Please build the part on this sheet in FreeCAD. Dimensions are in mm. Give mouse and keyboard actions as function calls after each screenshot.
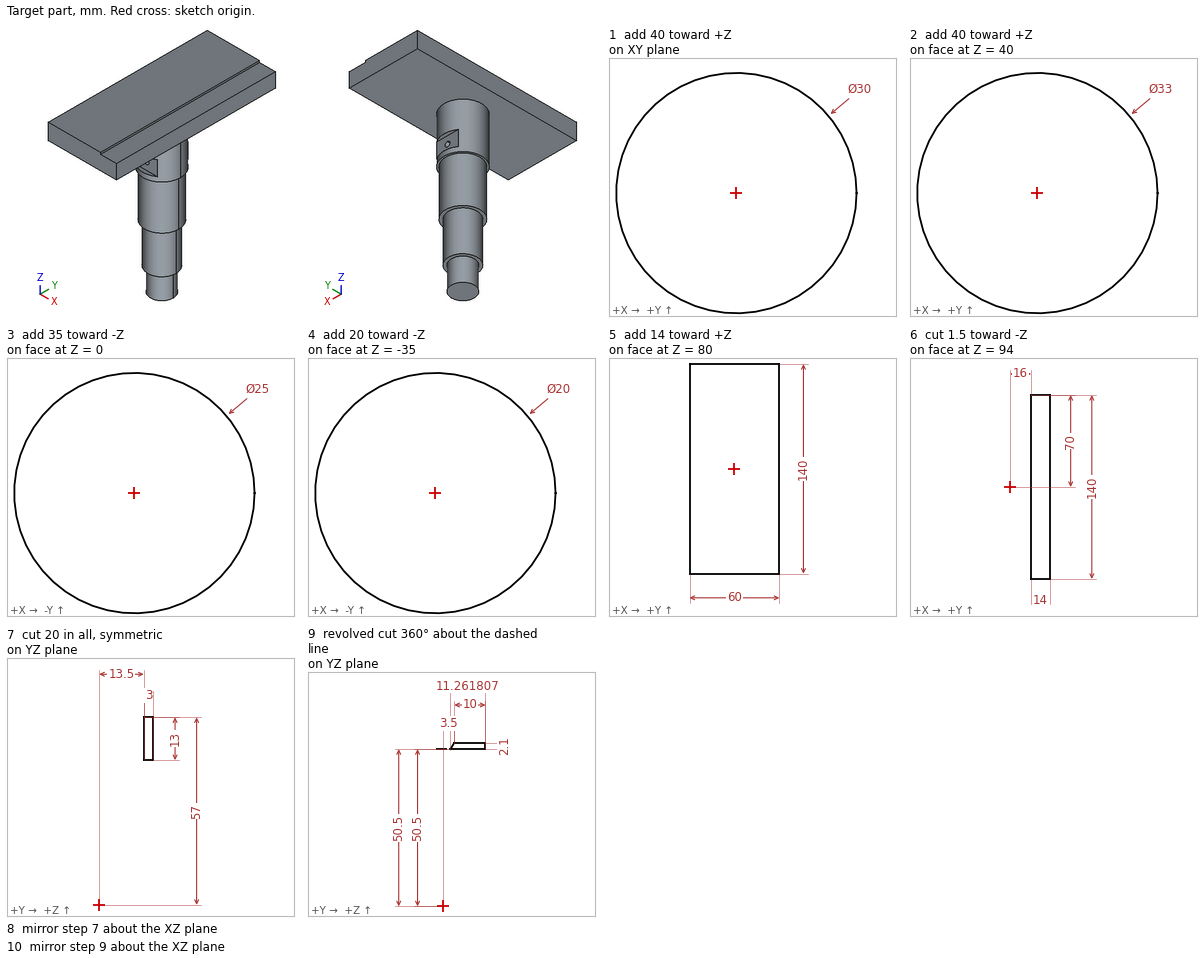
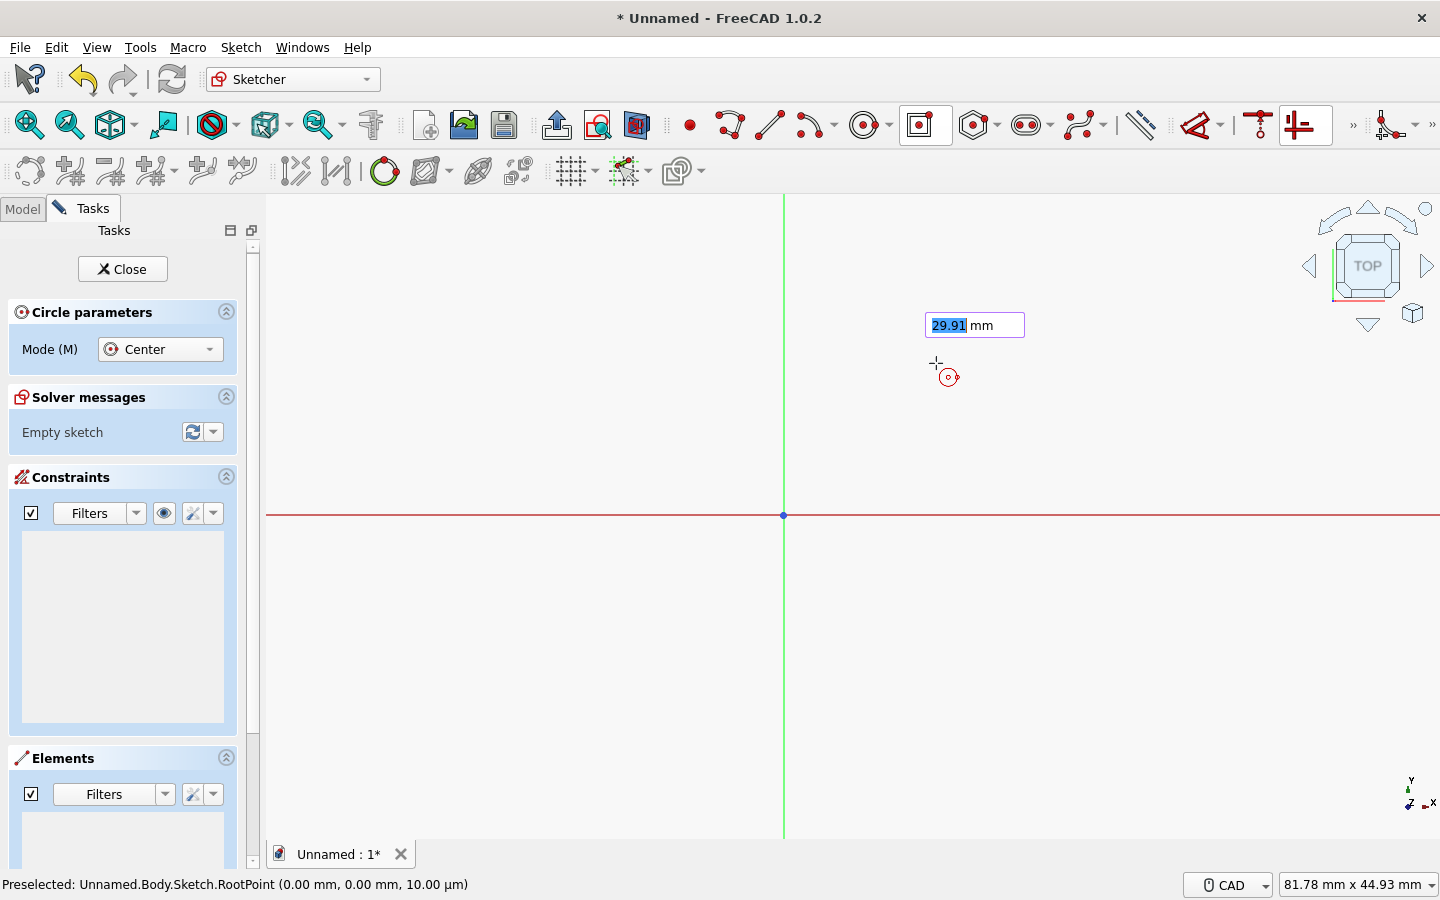
text(30)
key(Return)
key(Escape)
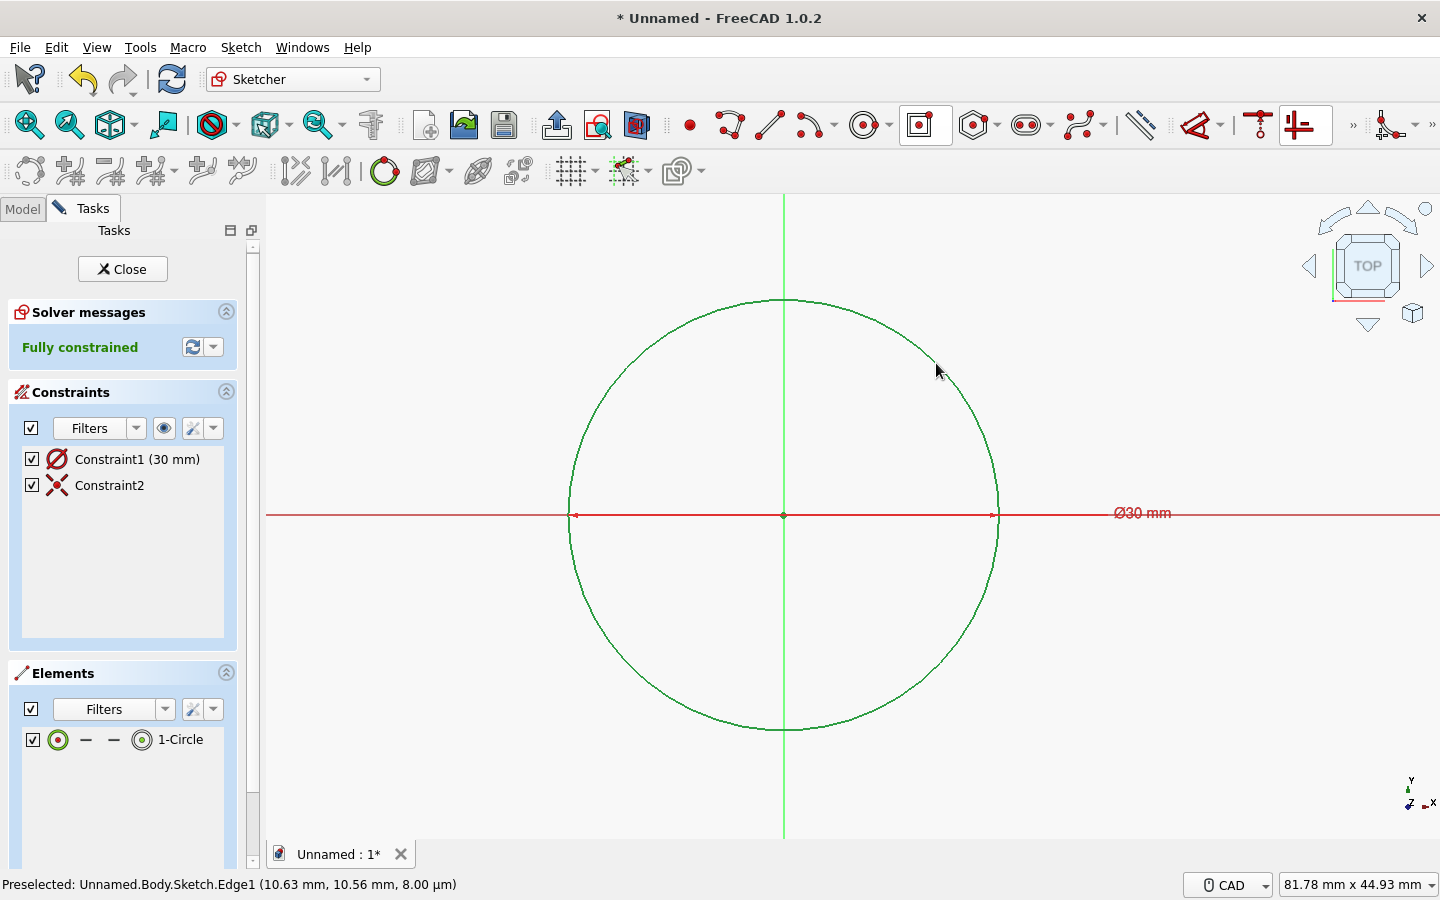
click(123, 269)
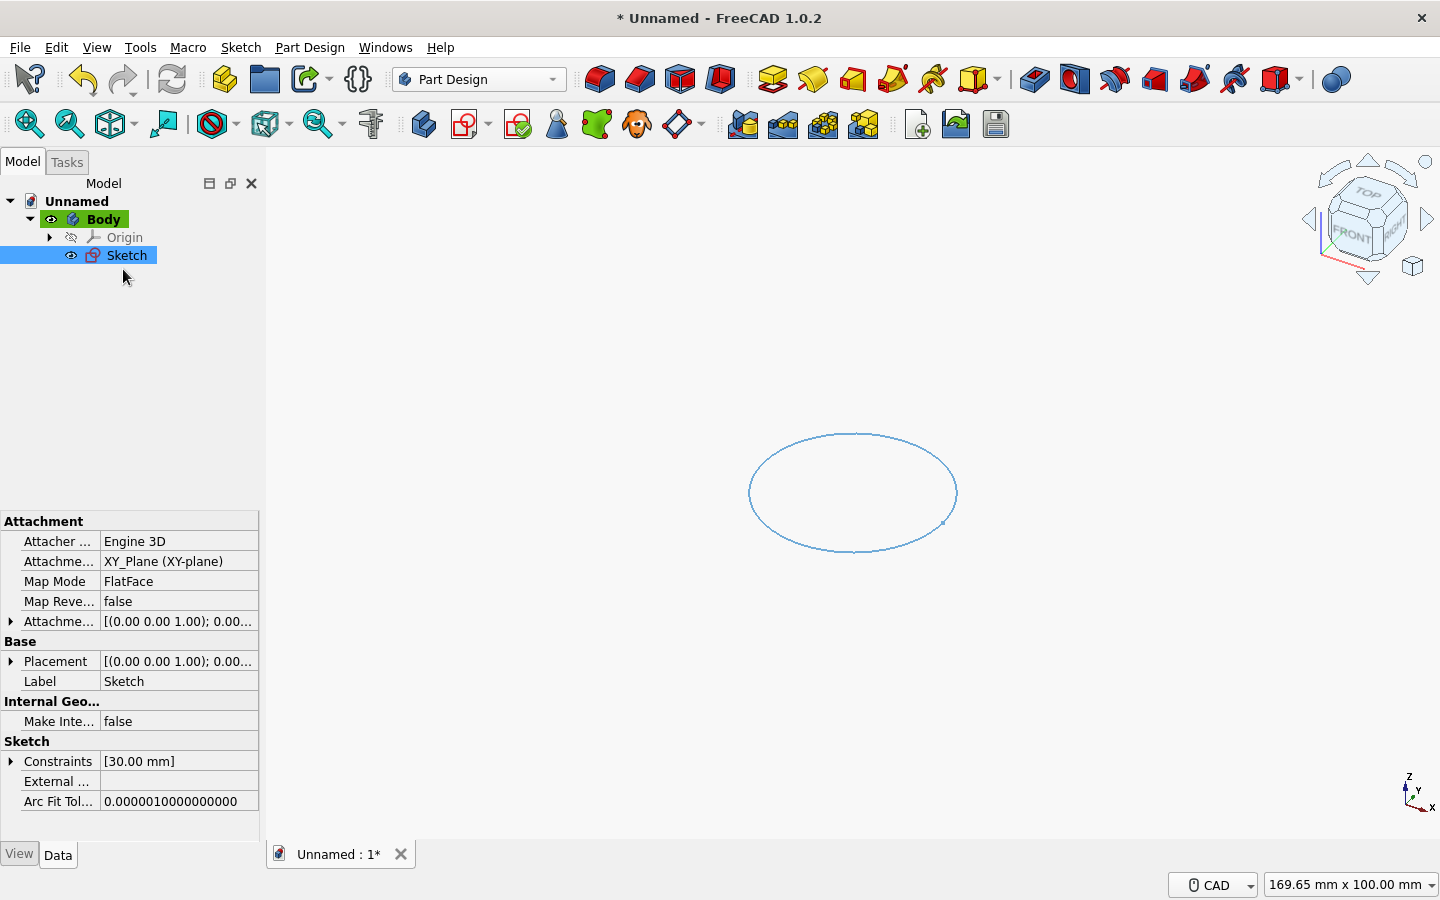
click(774, 80)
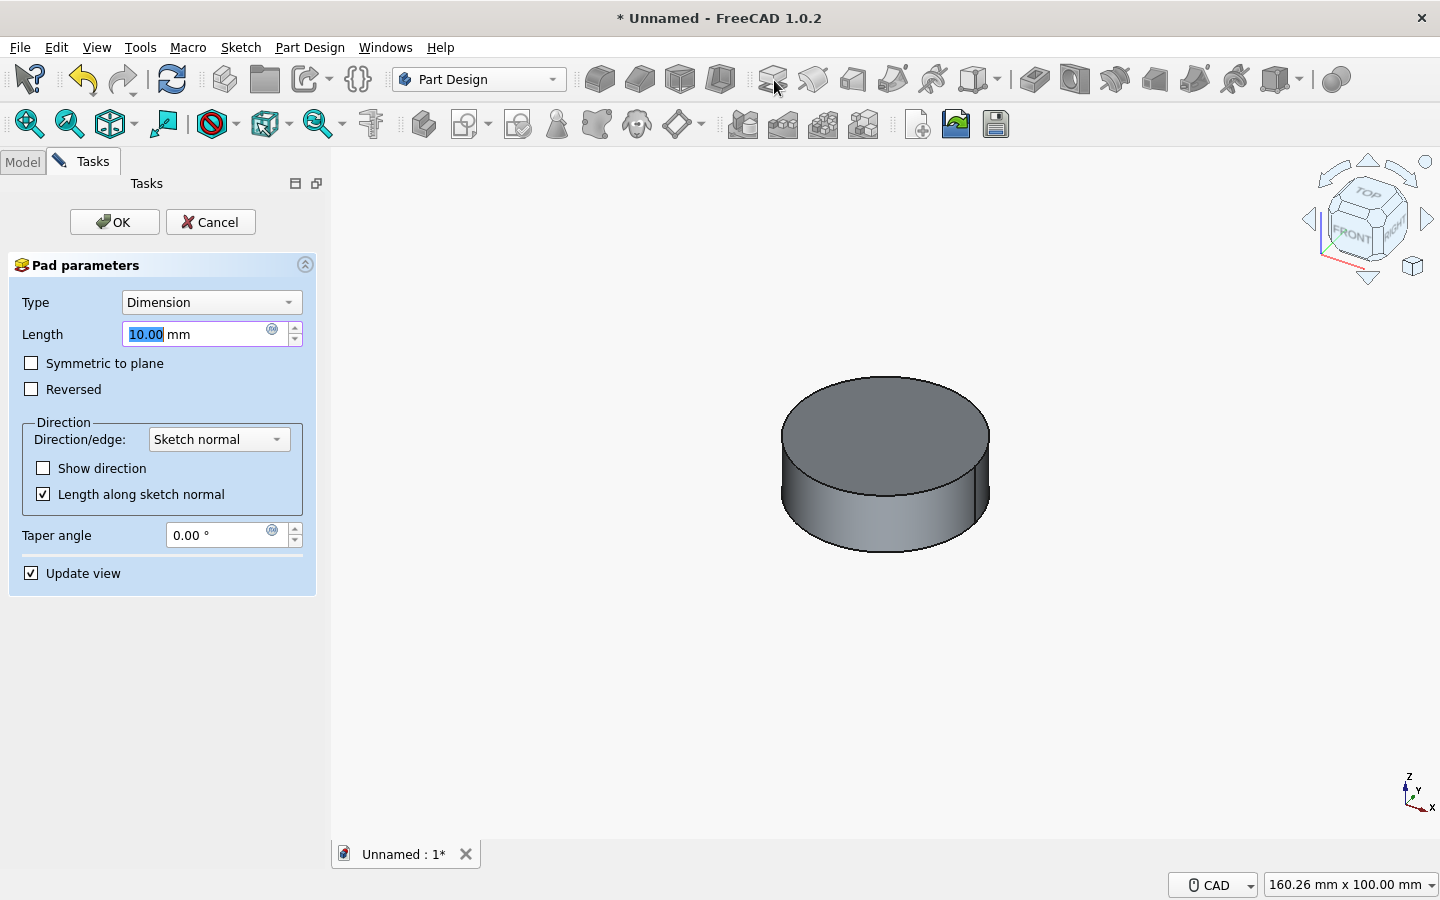
text(40)
key(Tab)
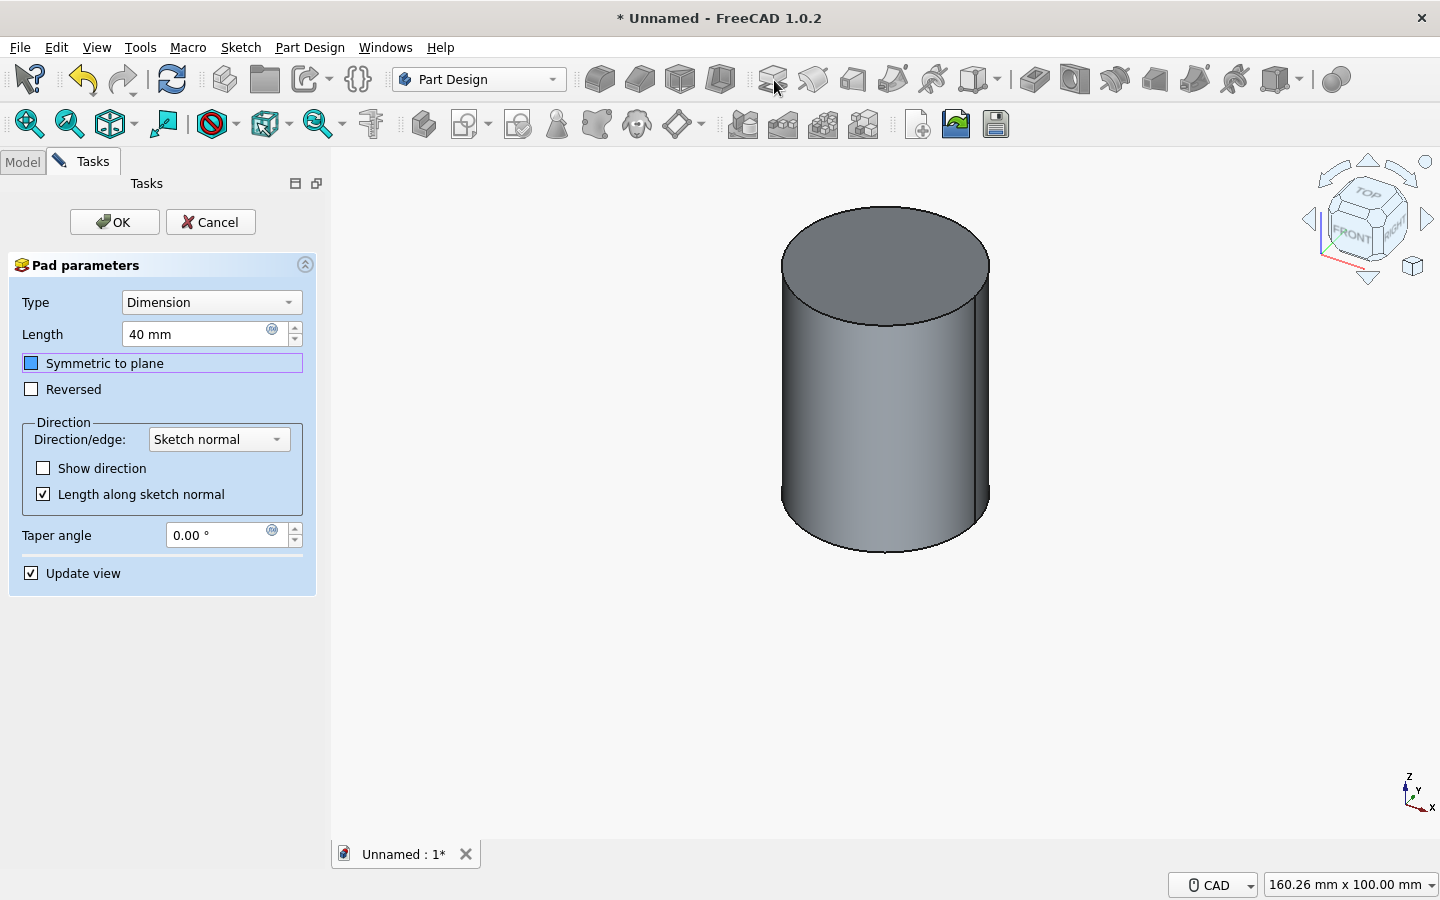
click(115, 222)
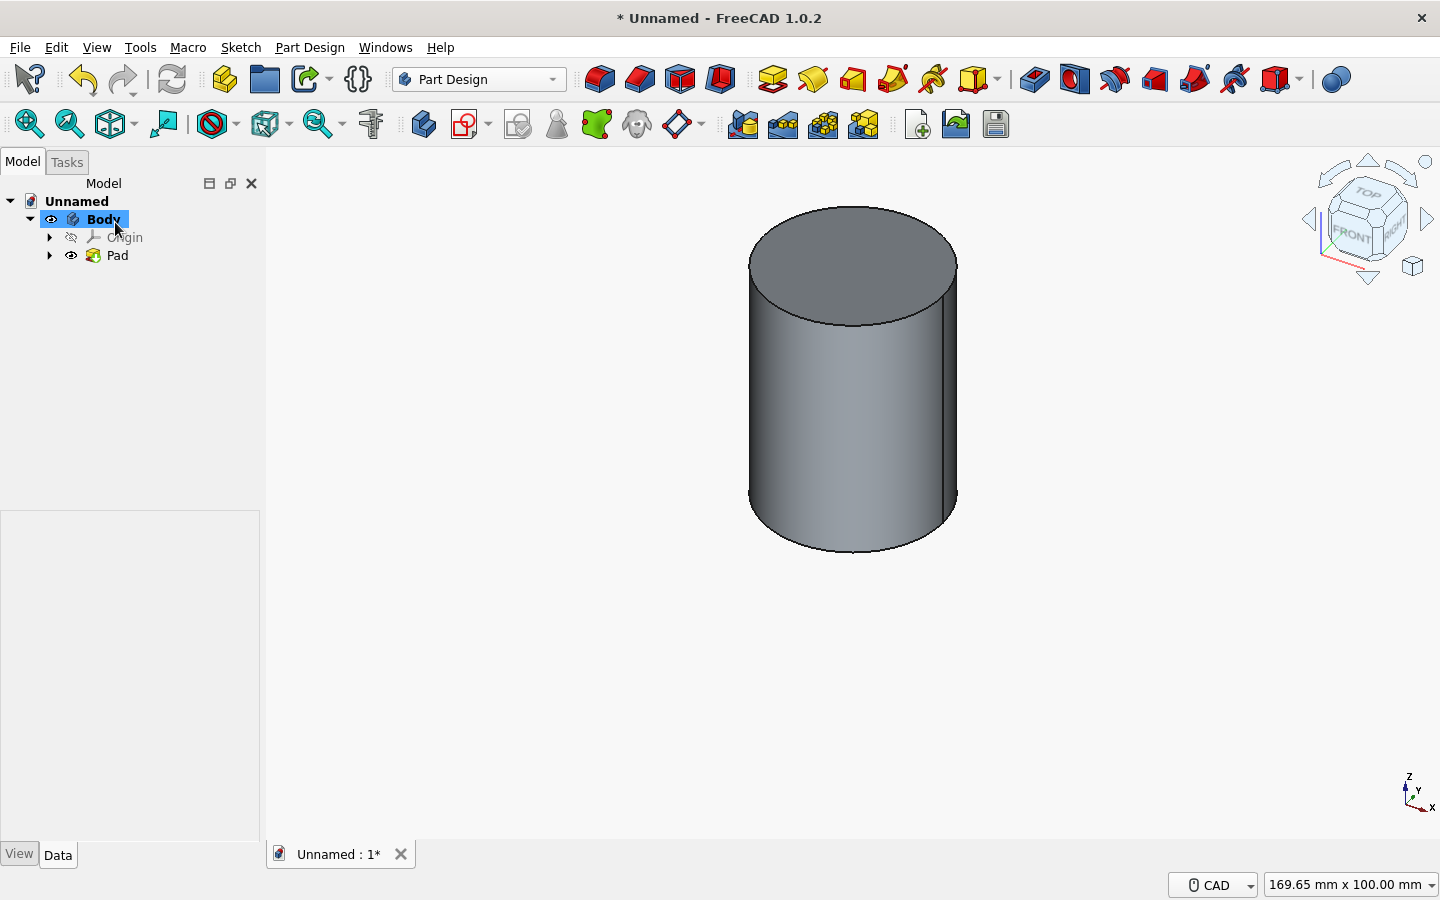
click(853, 265)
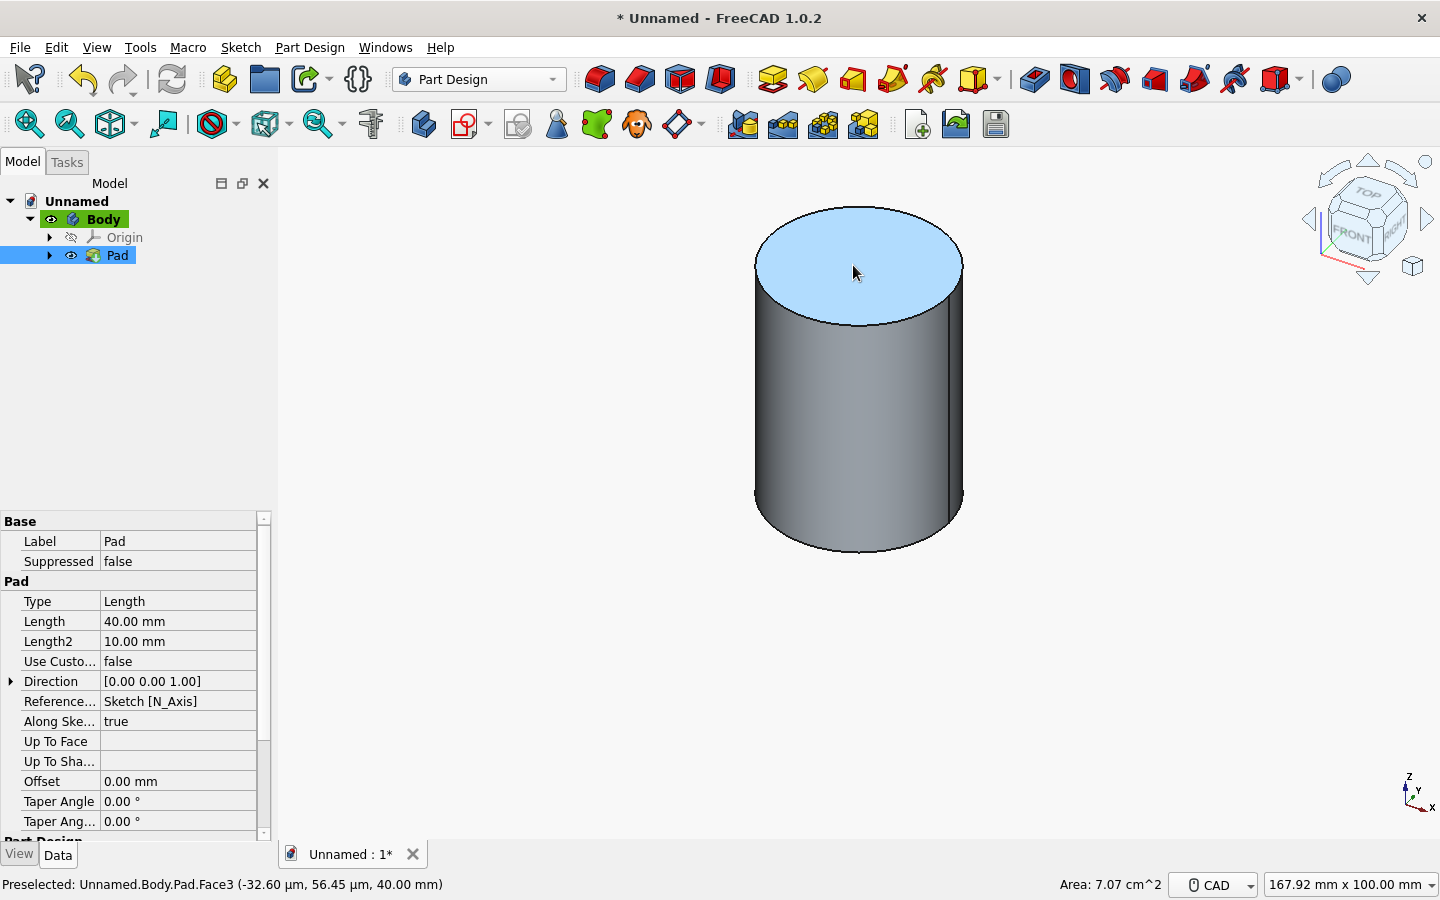
click(464, 124)